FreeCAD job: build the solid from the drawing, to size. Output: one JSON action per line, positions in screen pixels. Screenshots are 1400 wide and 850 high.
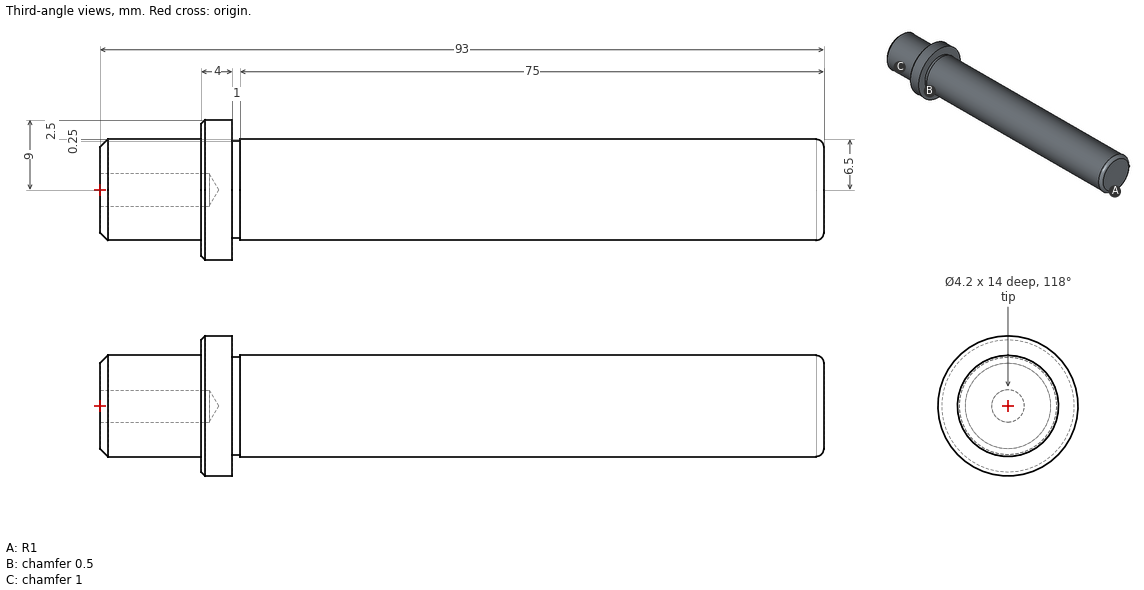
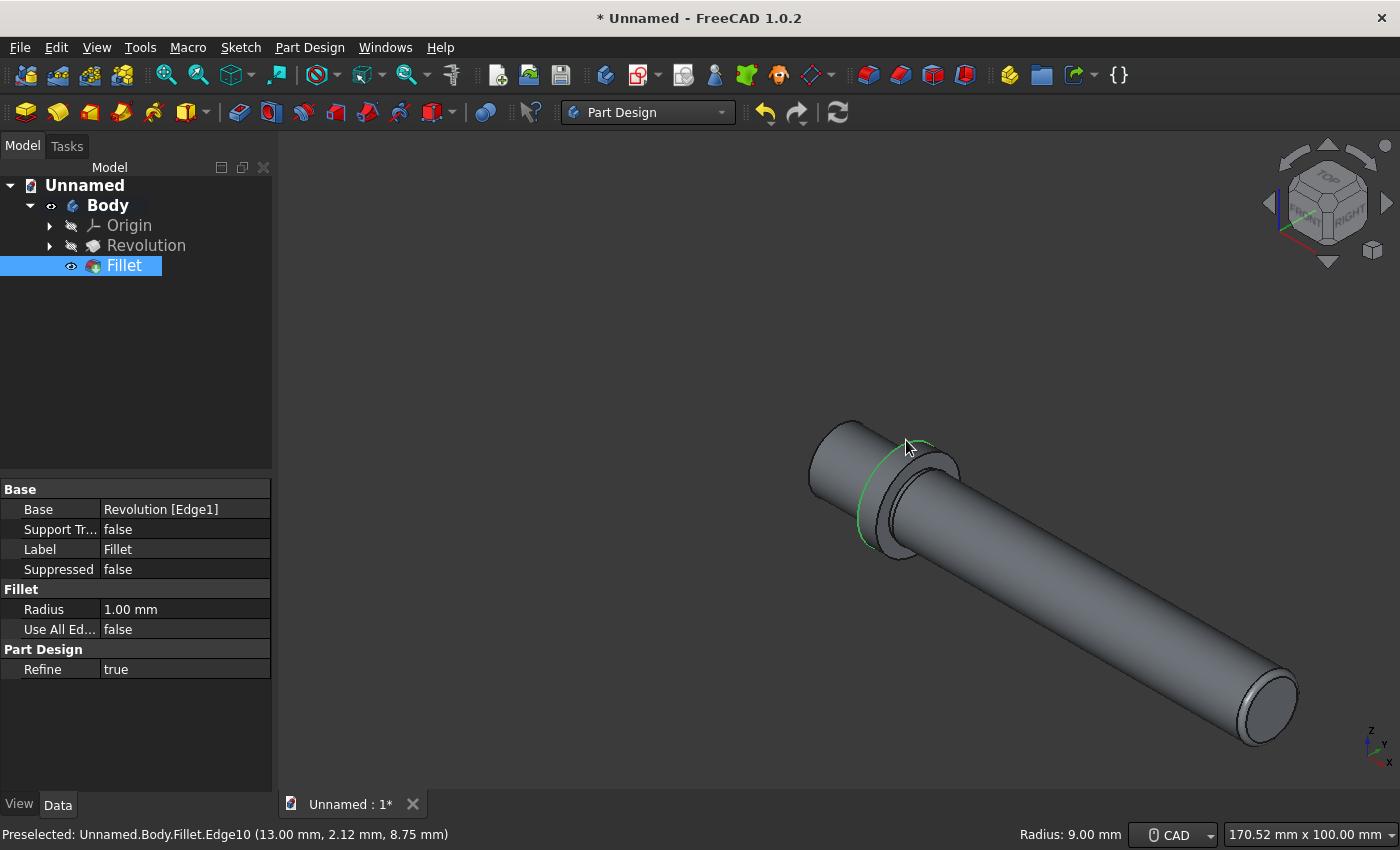
{"action": "left_click", "coordinate": [902, 76]}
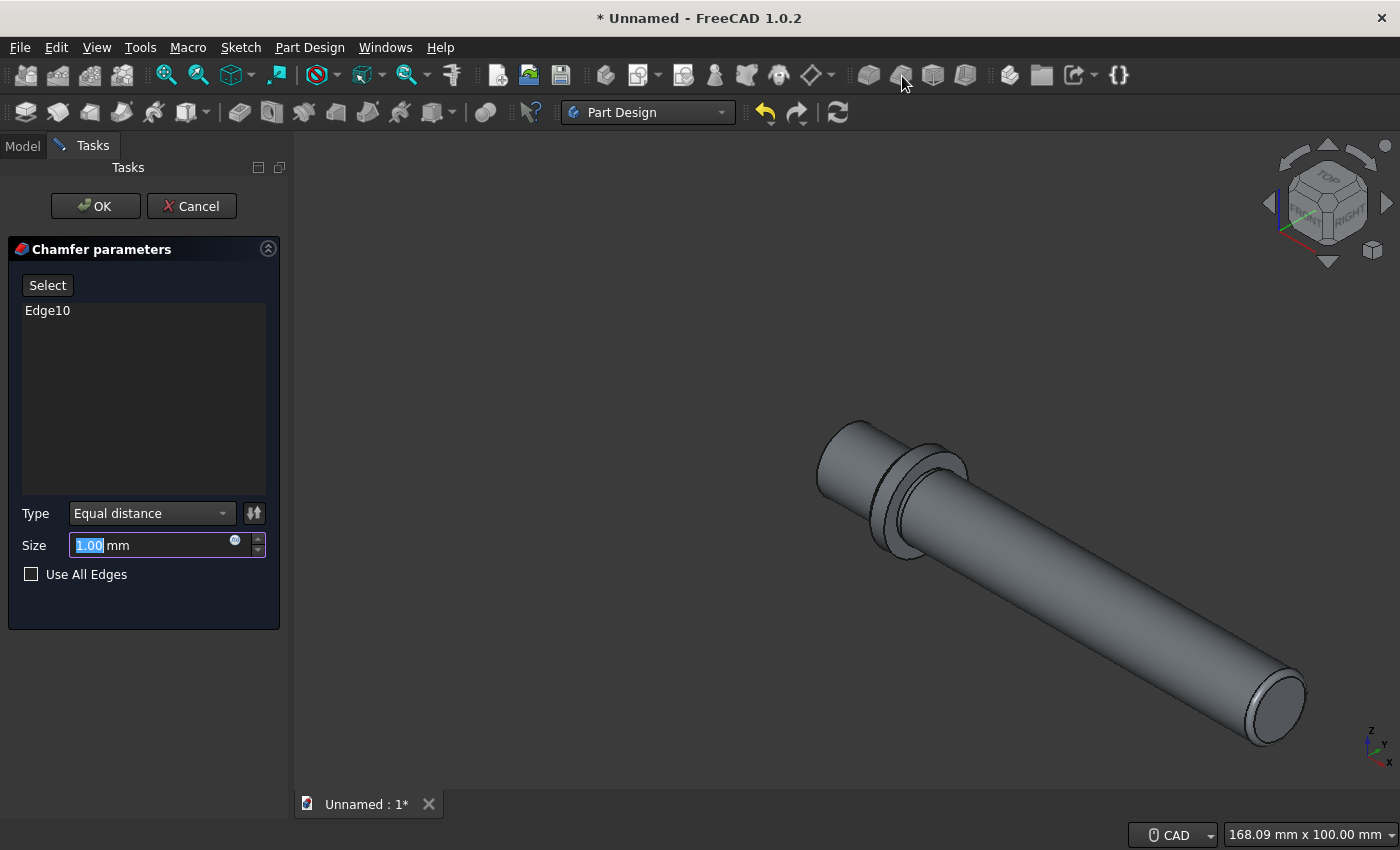
{"action": "type", "text": "0.5"}
{"action": "key", "text": "Tab"}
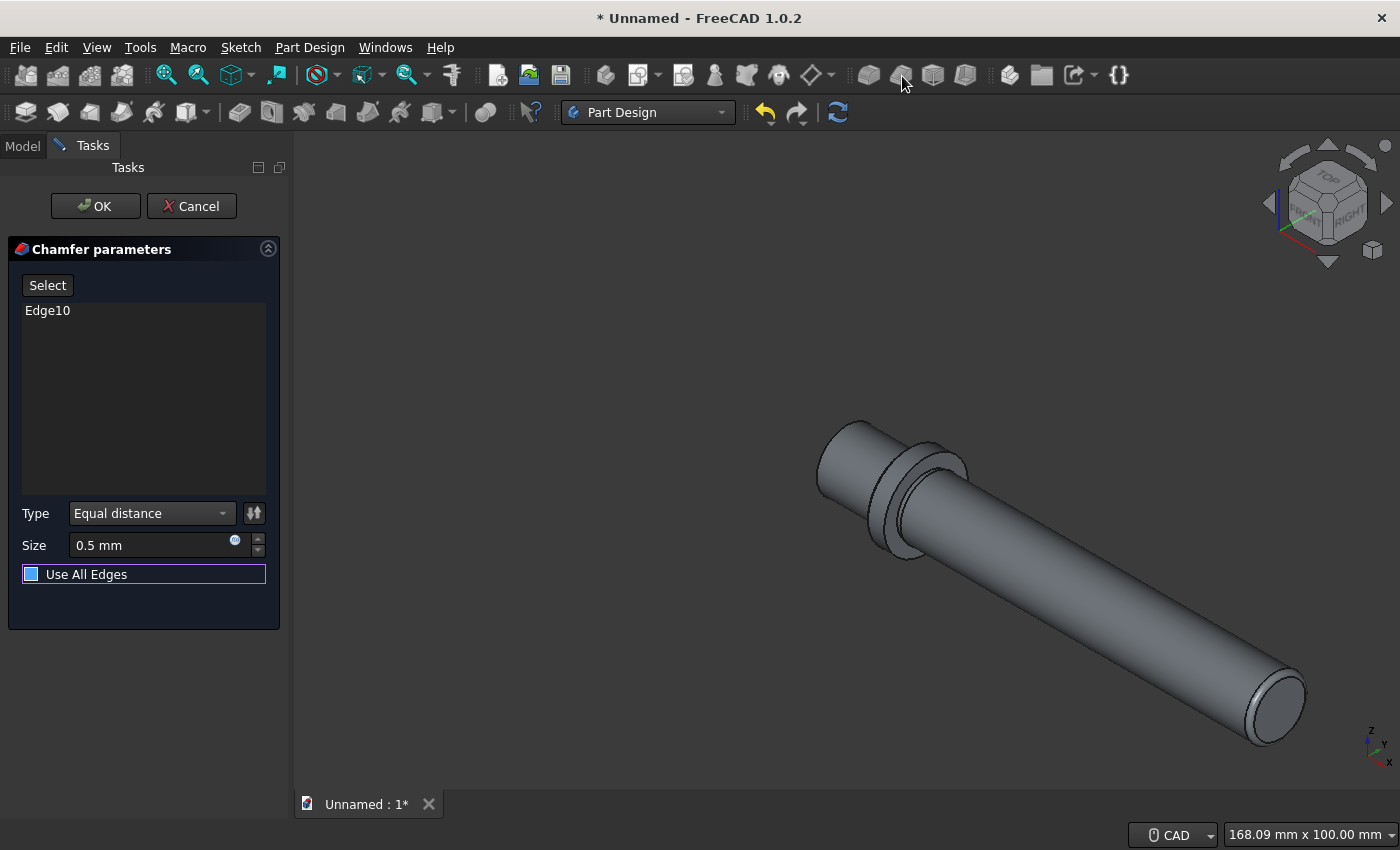
{"action": "left_click", "coordinate": [96, 206]}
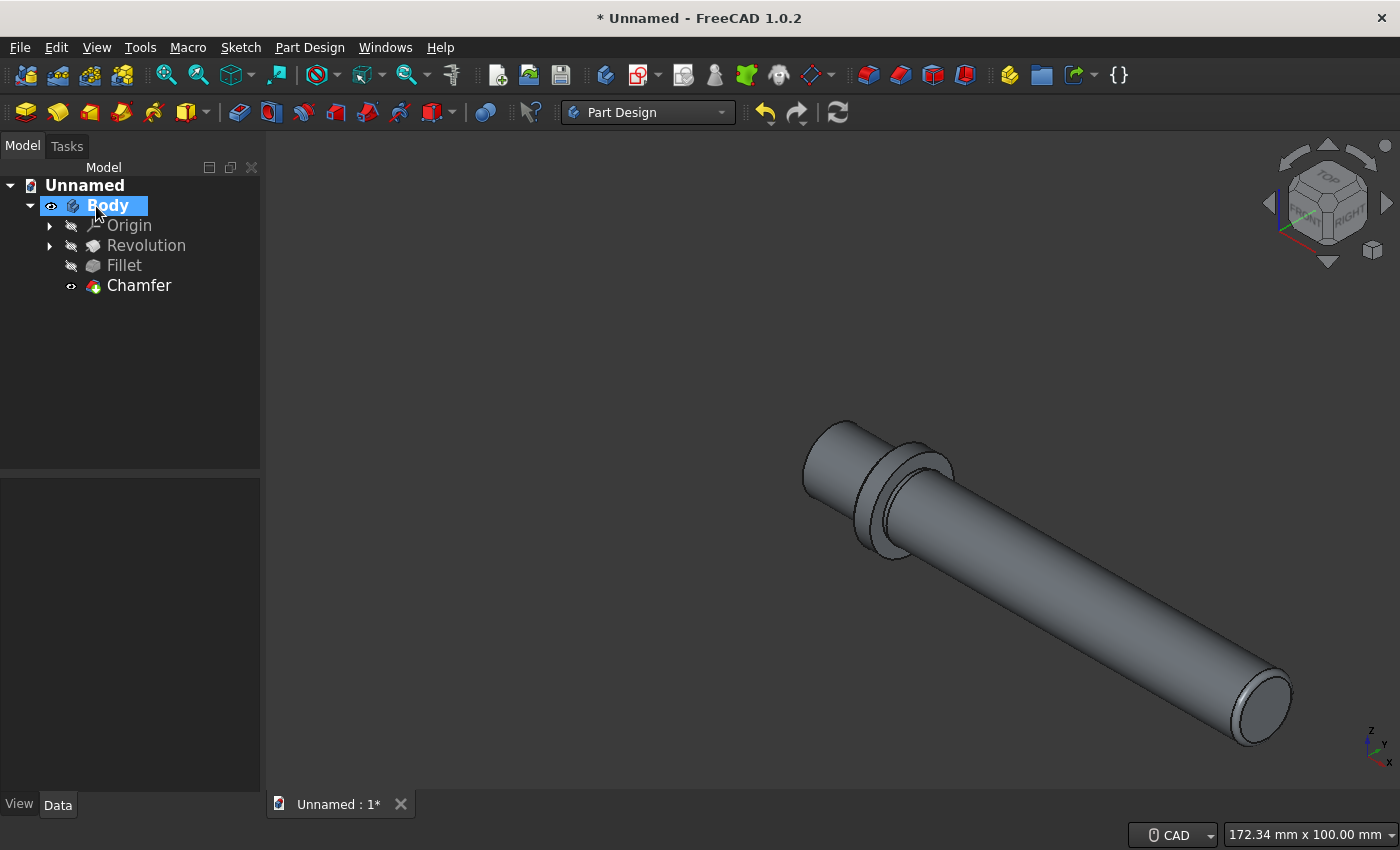
{"action": "left_click", "coordinate": [842, 420]}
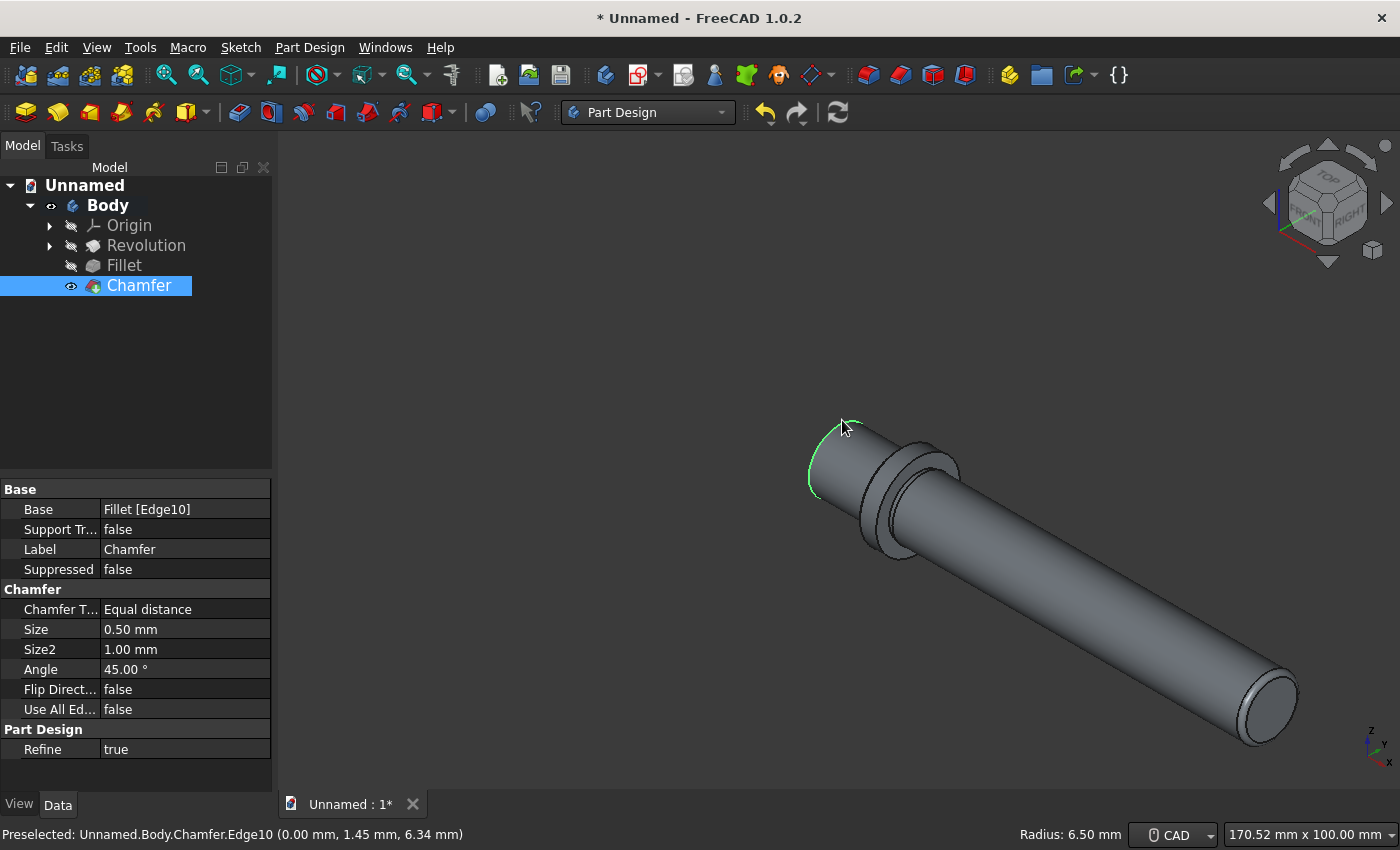
{"action": "left_click", "coordinate": [902, 76]}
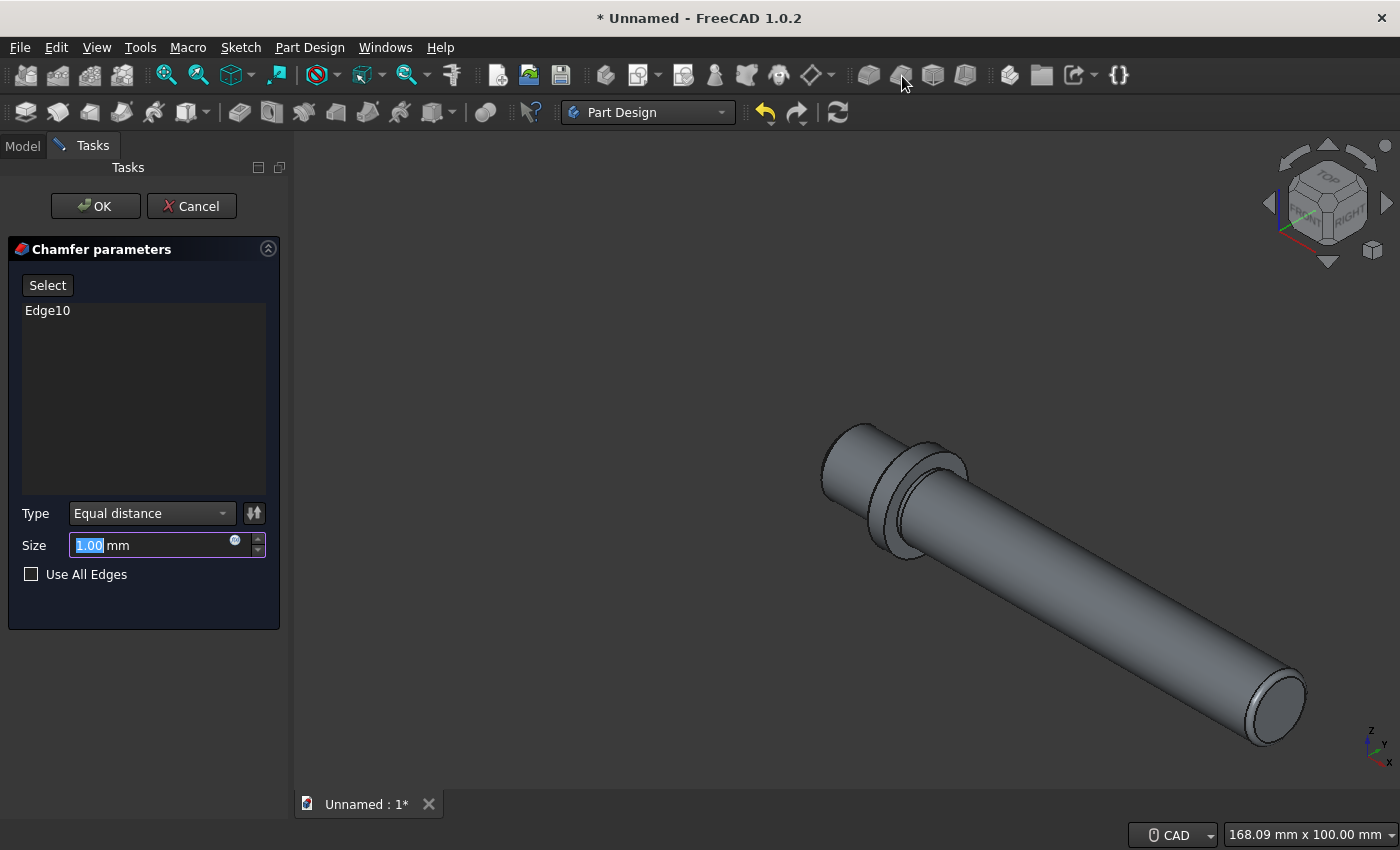
{"action": "type", "text": "1"}
{"action": "key", "text": "Tab"}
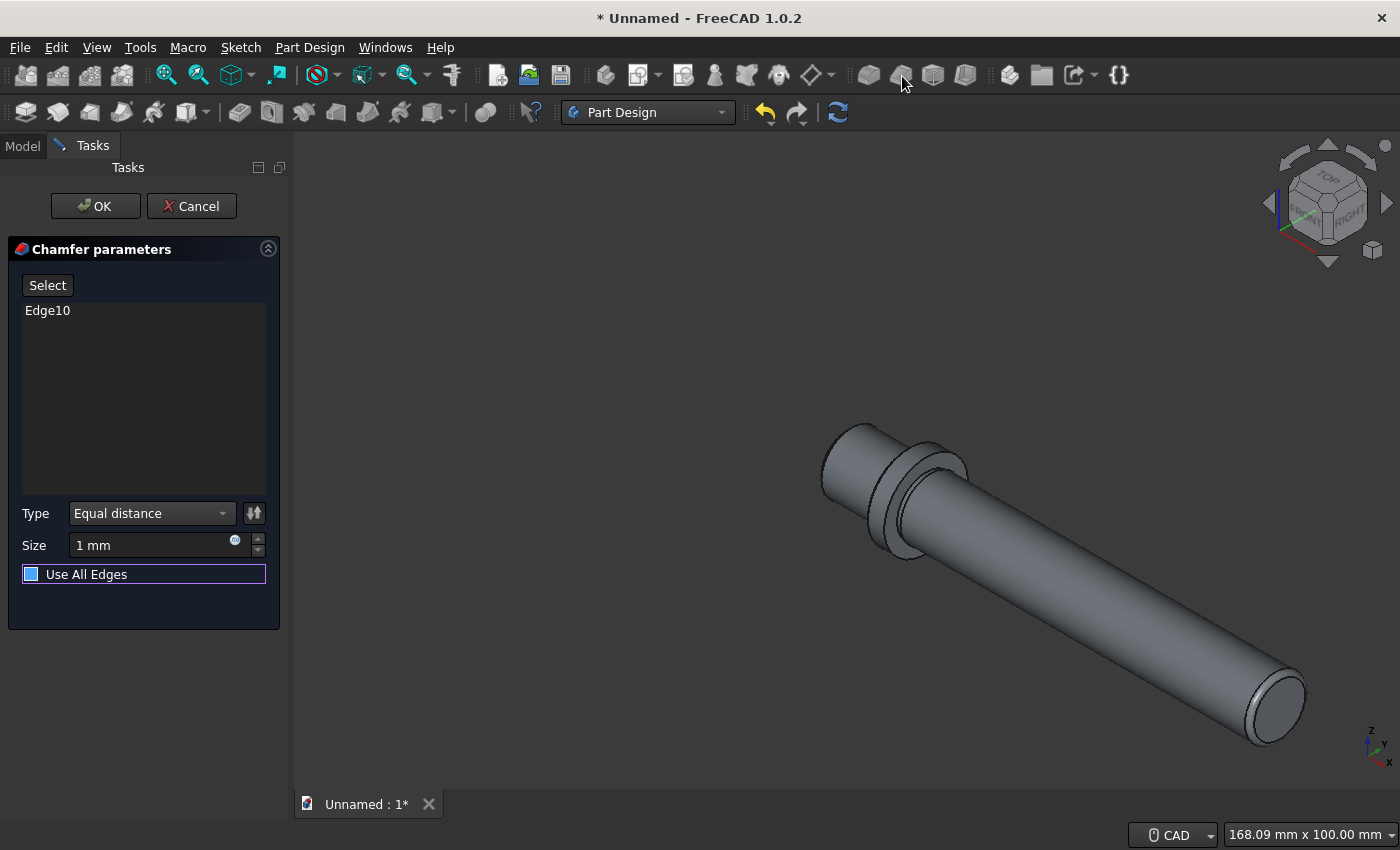
{"action": "left_click", "coordinate": [96, 206]}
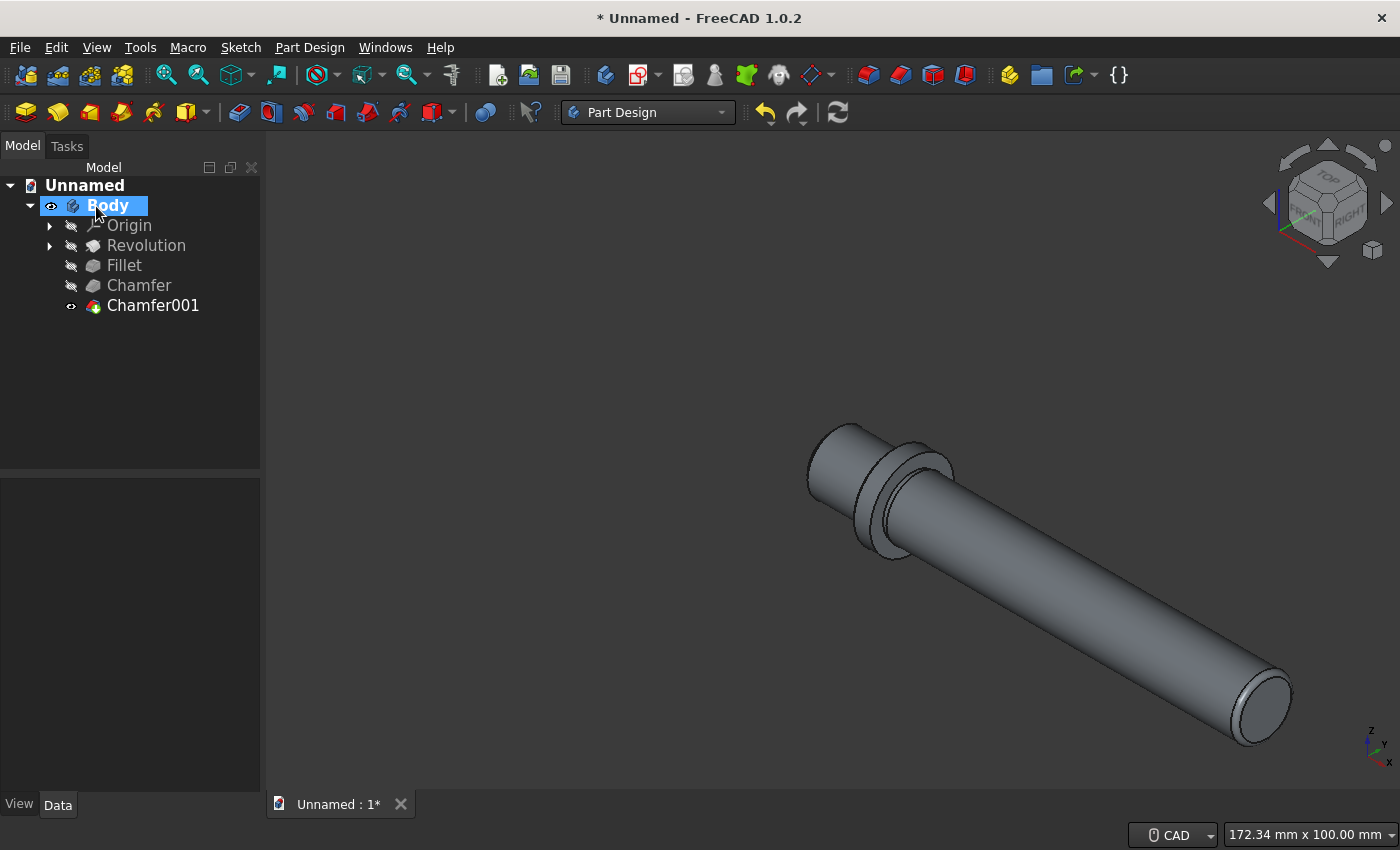
{"action": "key", "text": "6"}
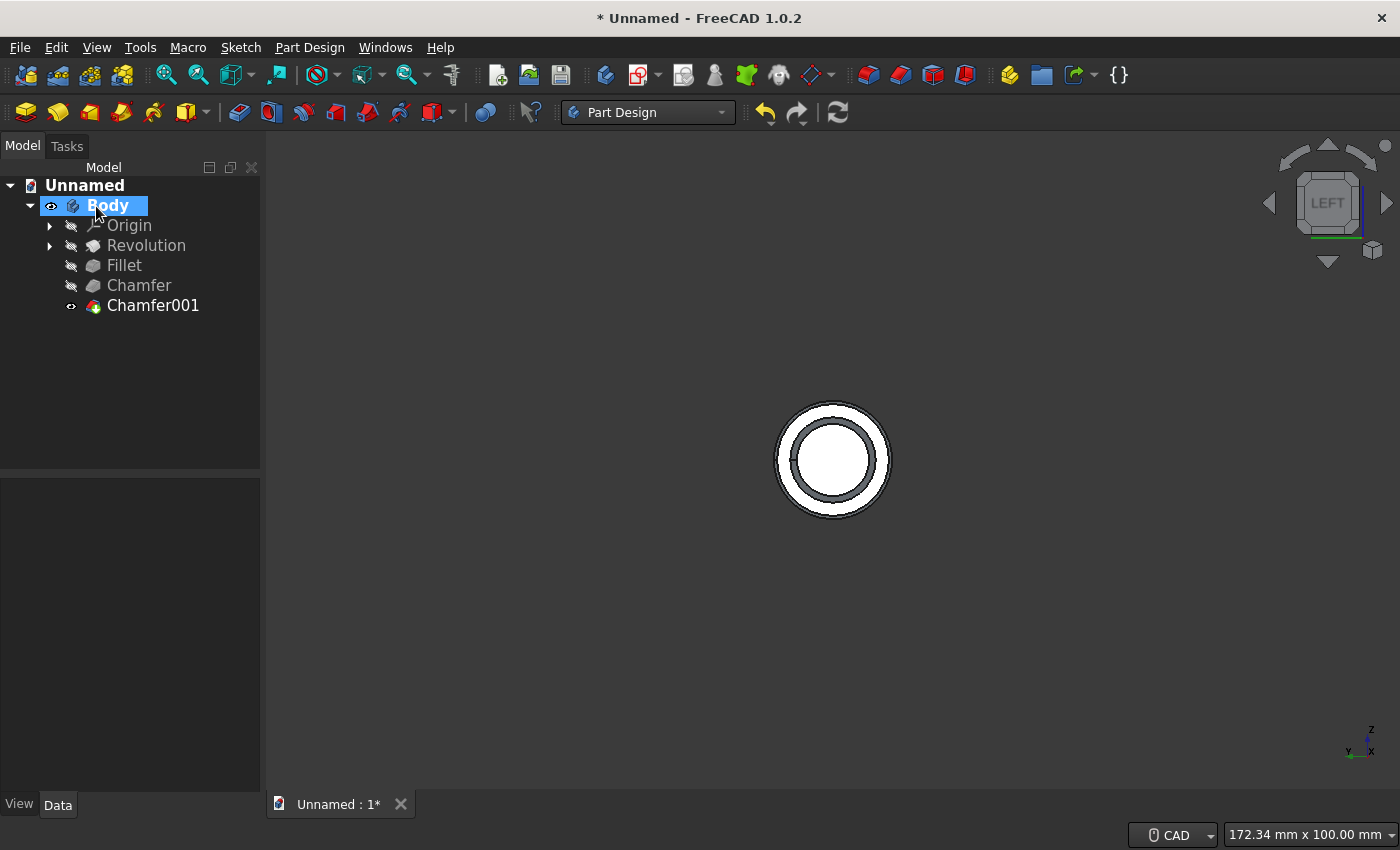
{"action": "key", "text": "v f"}